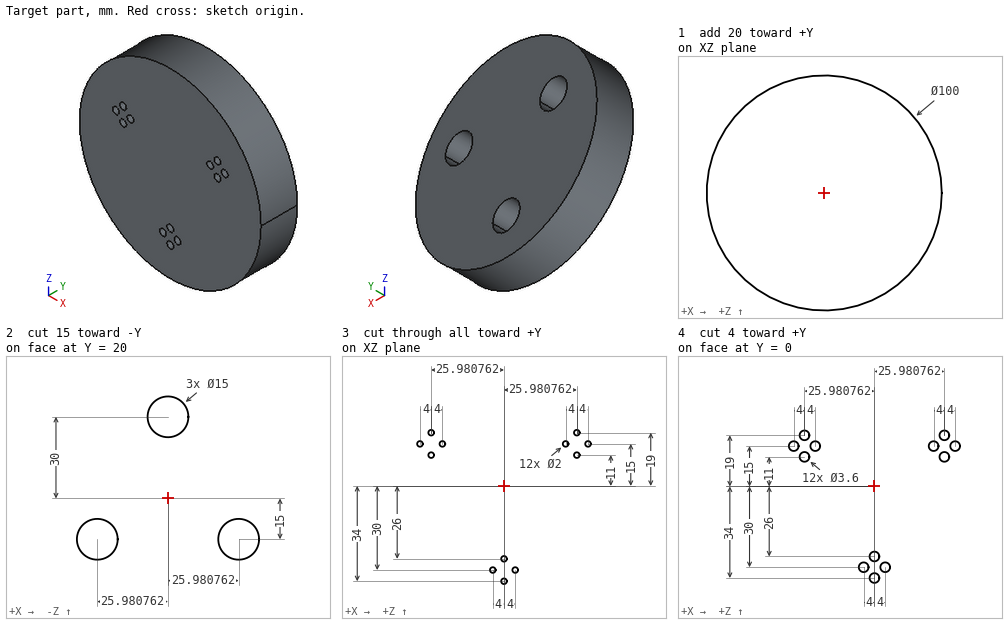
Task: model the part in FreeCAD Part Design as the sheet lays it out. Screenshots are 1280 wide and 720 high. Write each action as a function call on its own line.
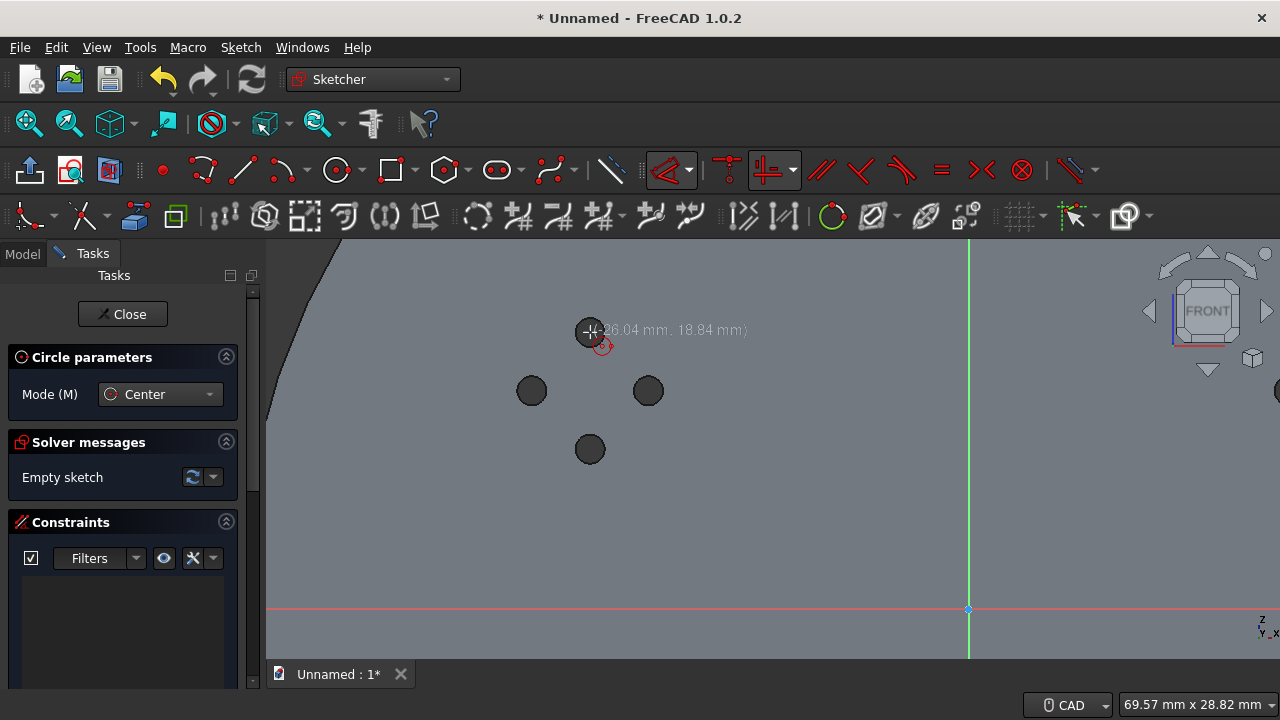
click(590, 333)
click(609, 314)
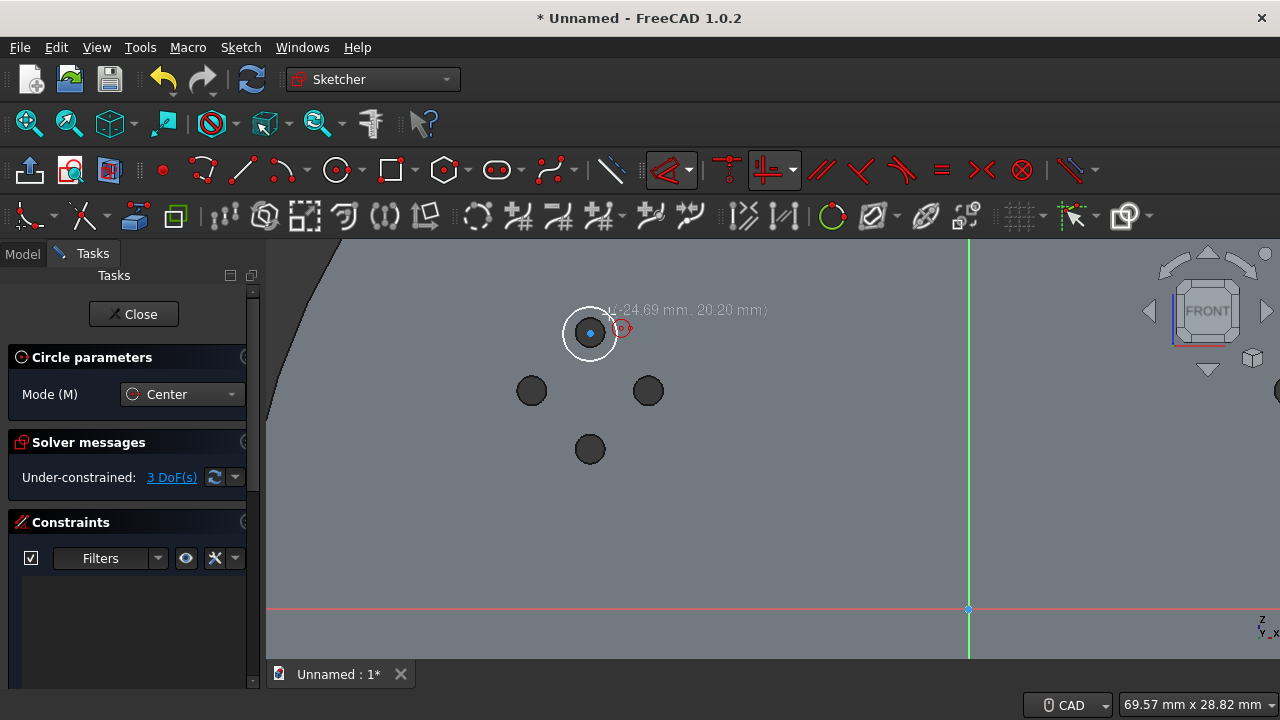
click(532, 391)
click(550, 372)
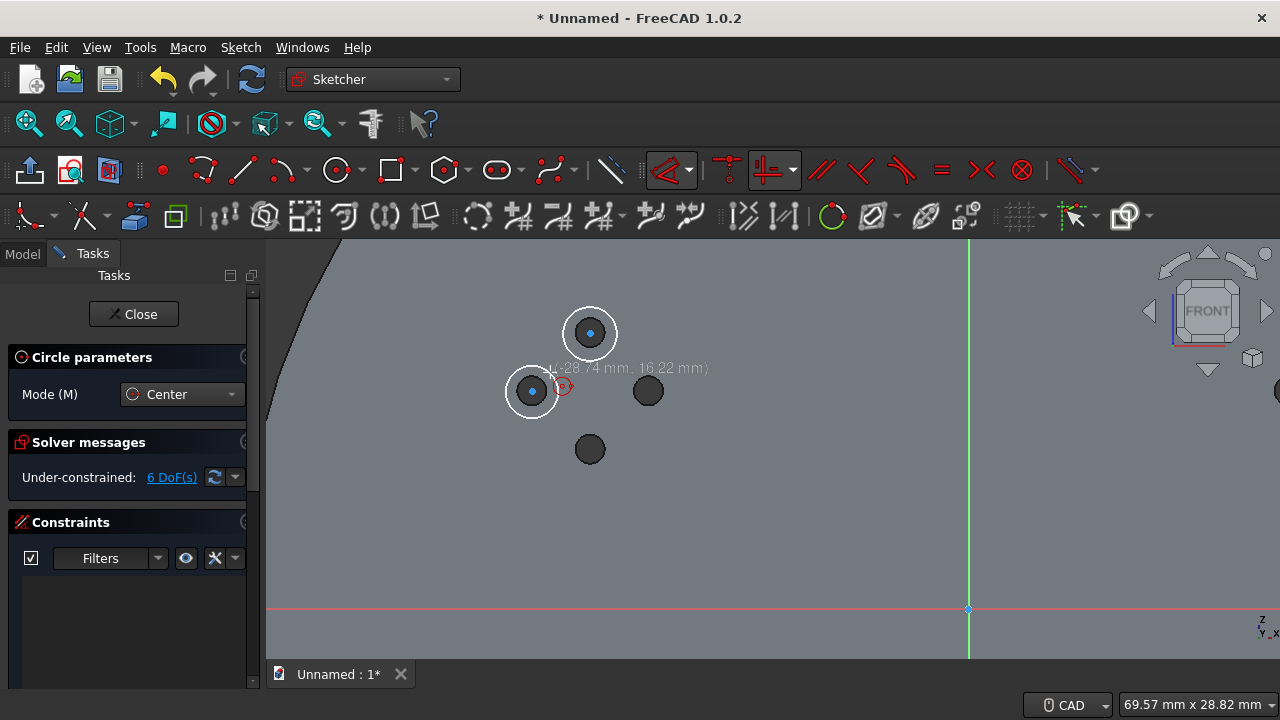
click(590, 449)
click(609, 431)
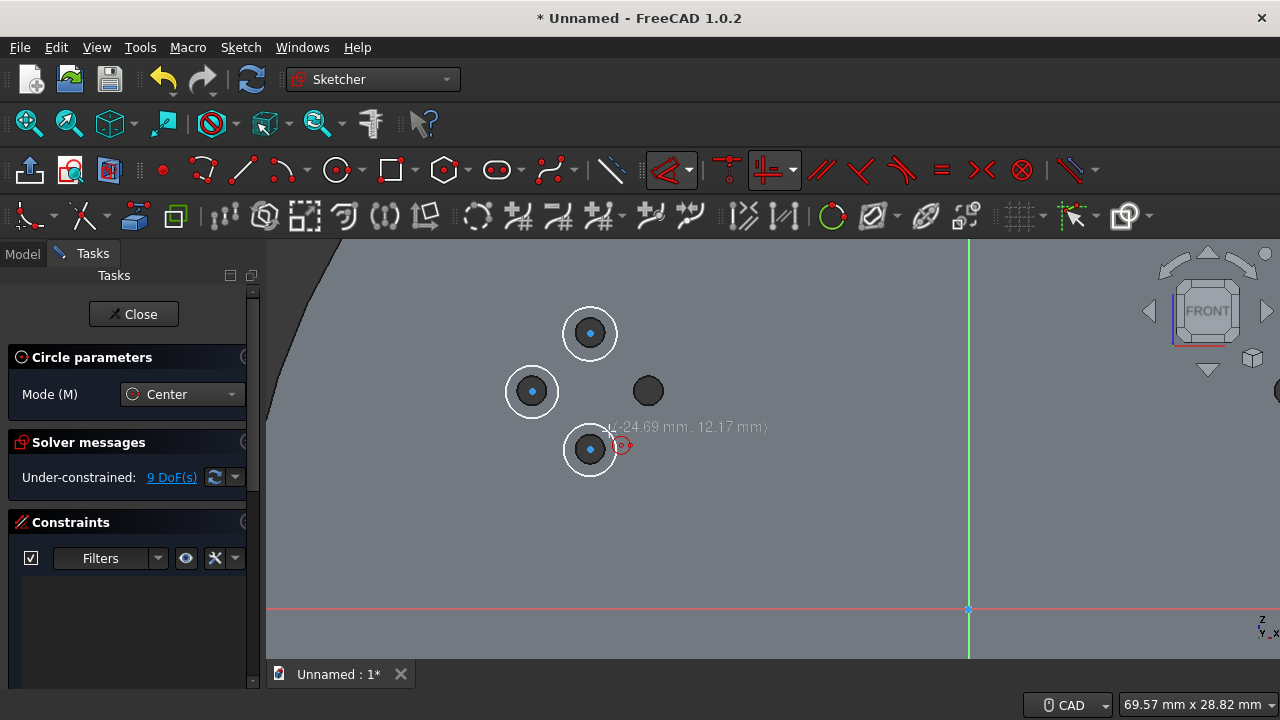
click(648, 391)
click(667, 372)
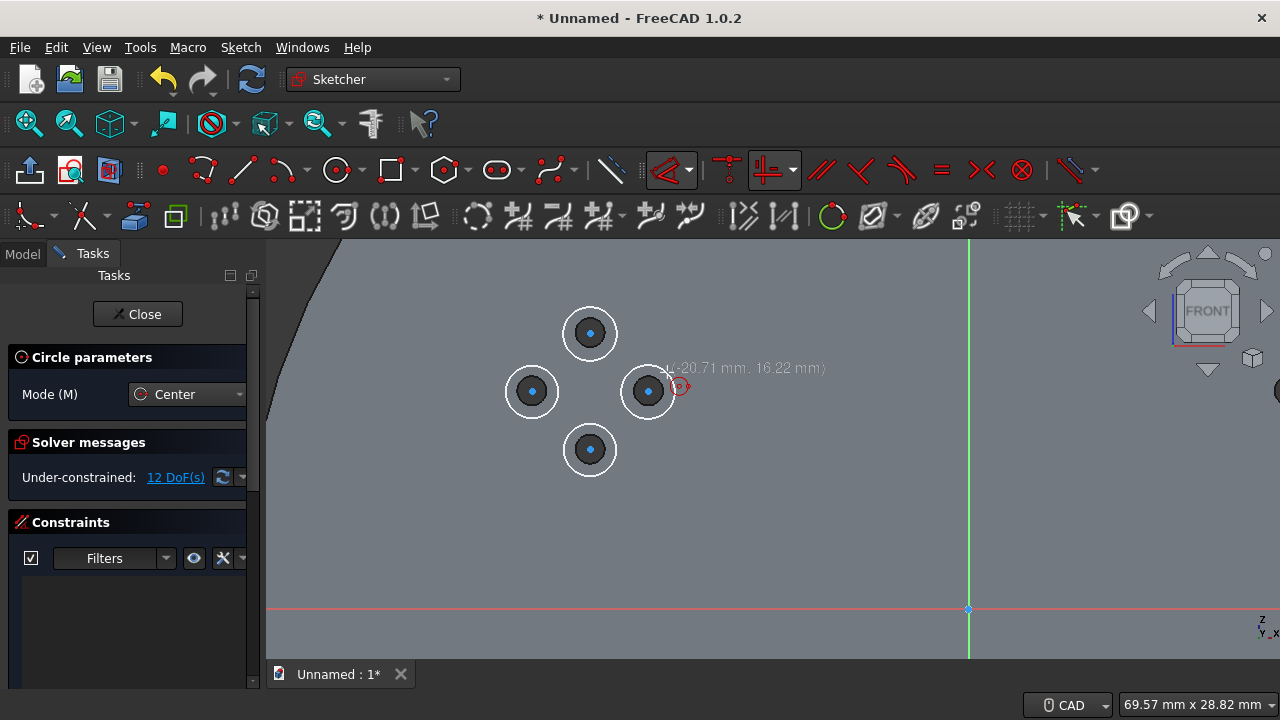
scroll(591, 333, down, 6)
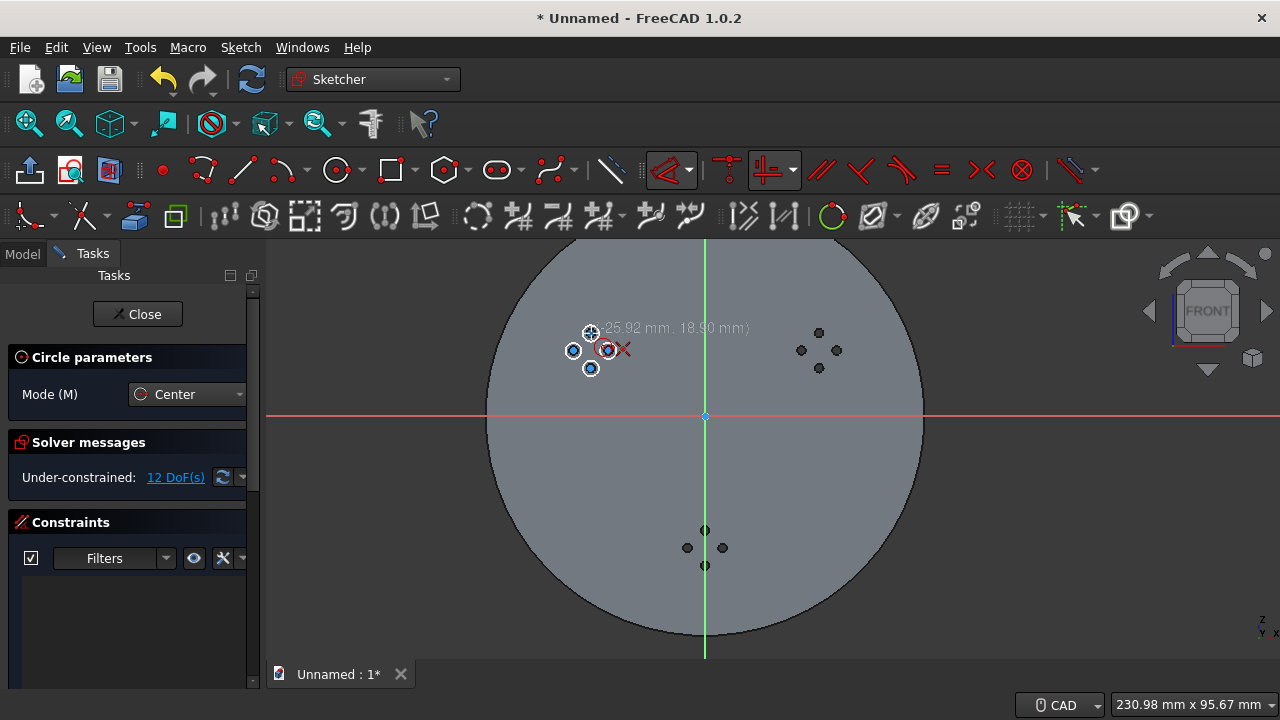
scroll(819, 333, up, 6)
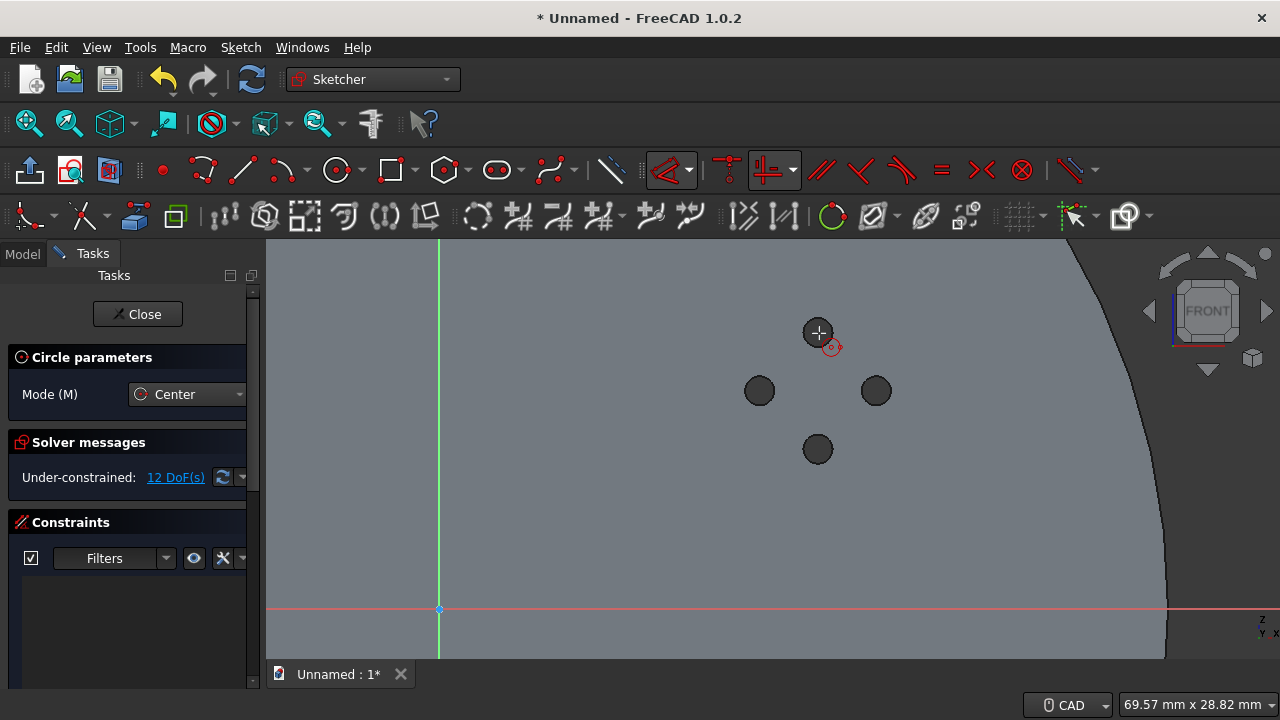
click(818, 333)
click(837, 314)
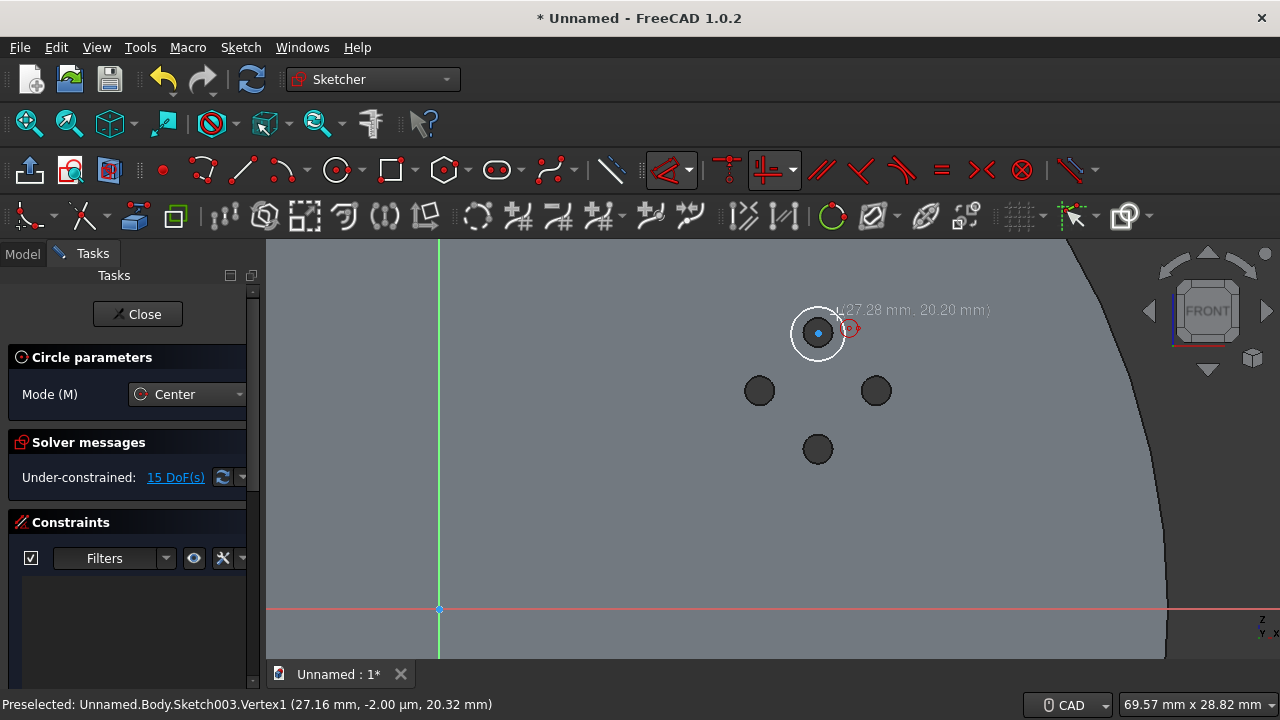
click(760, 391)
click(778, 372)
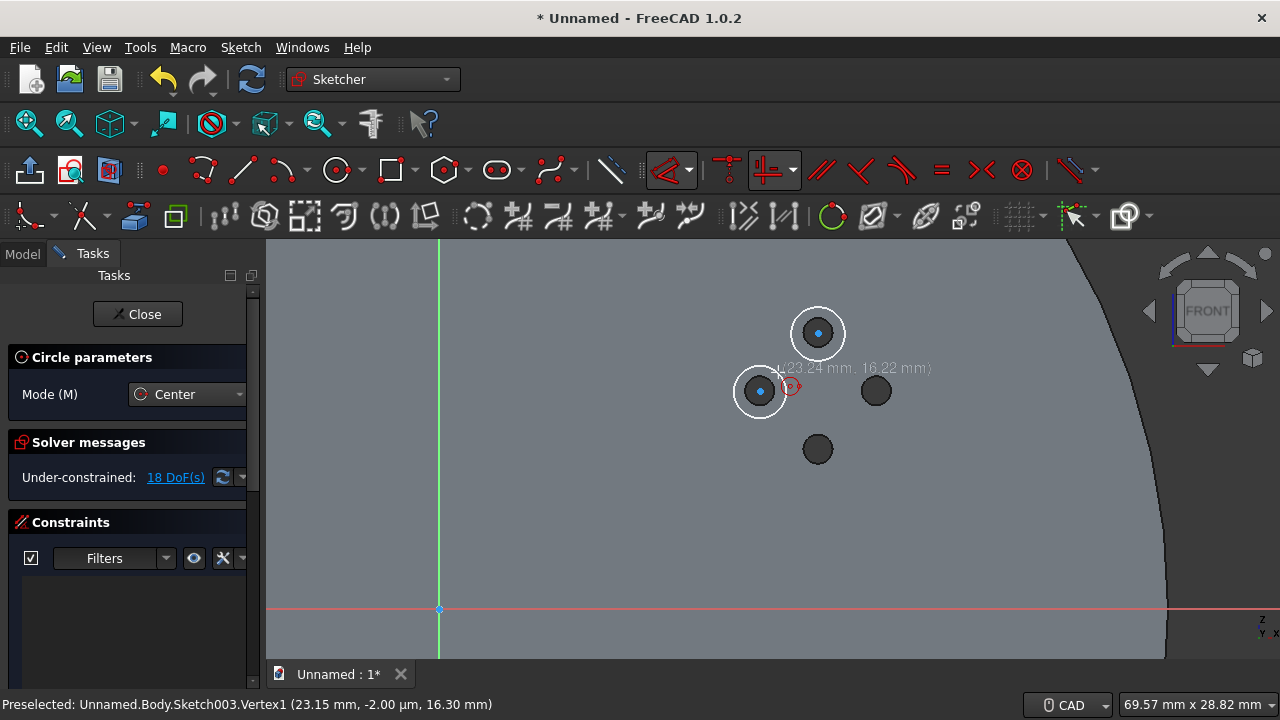
click(818, 449)
click(837, 431)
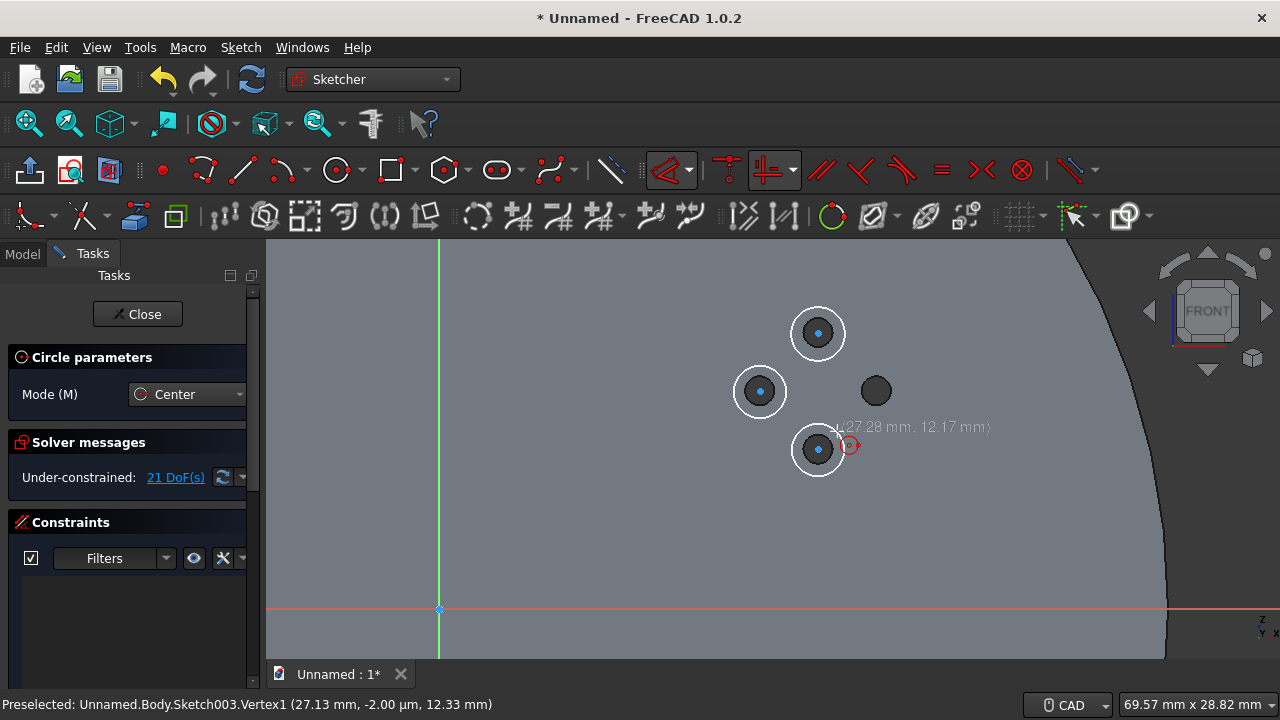
click(876, 391)
click(895, 372)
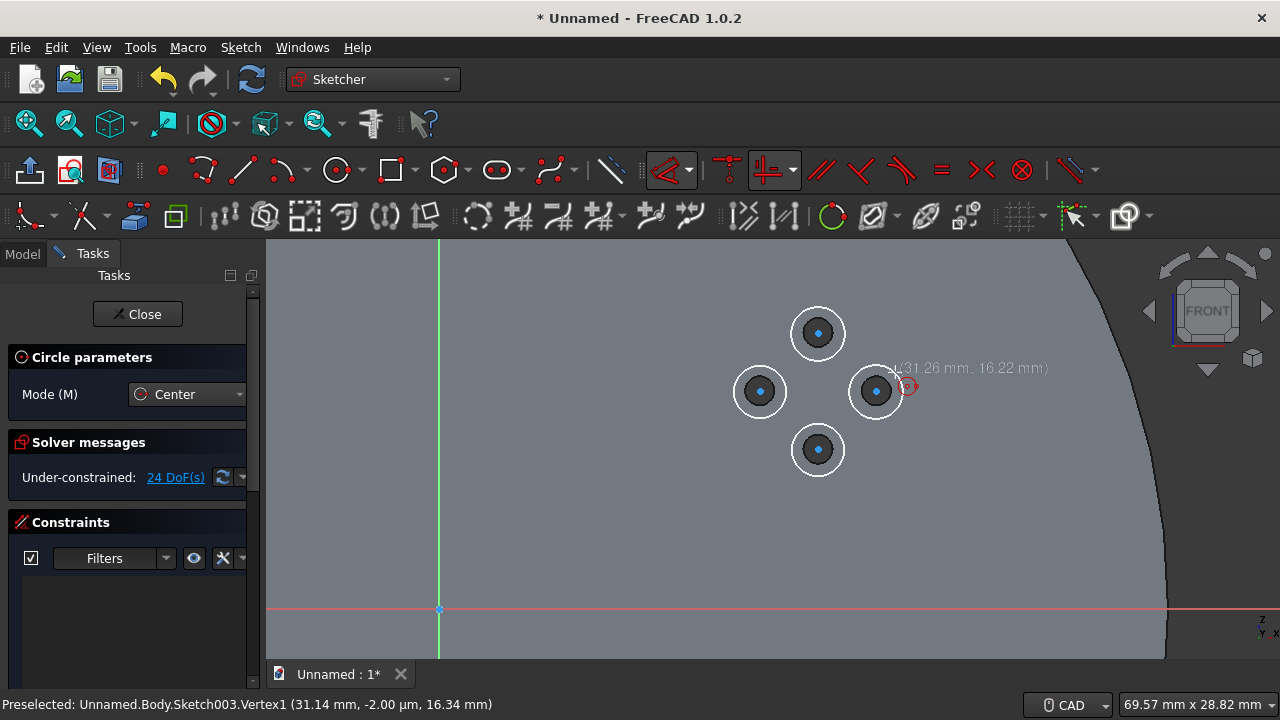
scroll(819, 333, down, 6)